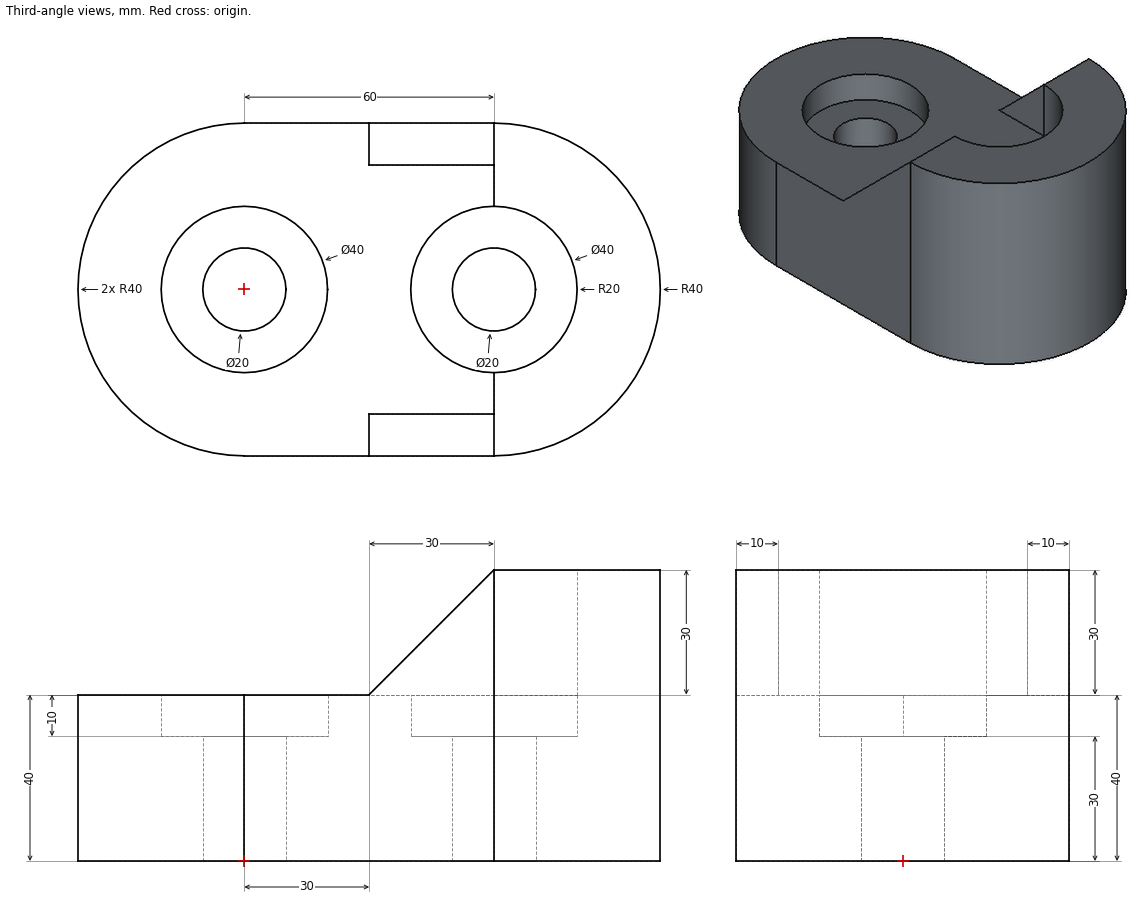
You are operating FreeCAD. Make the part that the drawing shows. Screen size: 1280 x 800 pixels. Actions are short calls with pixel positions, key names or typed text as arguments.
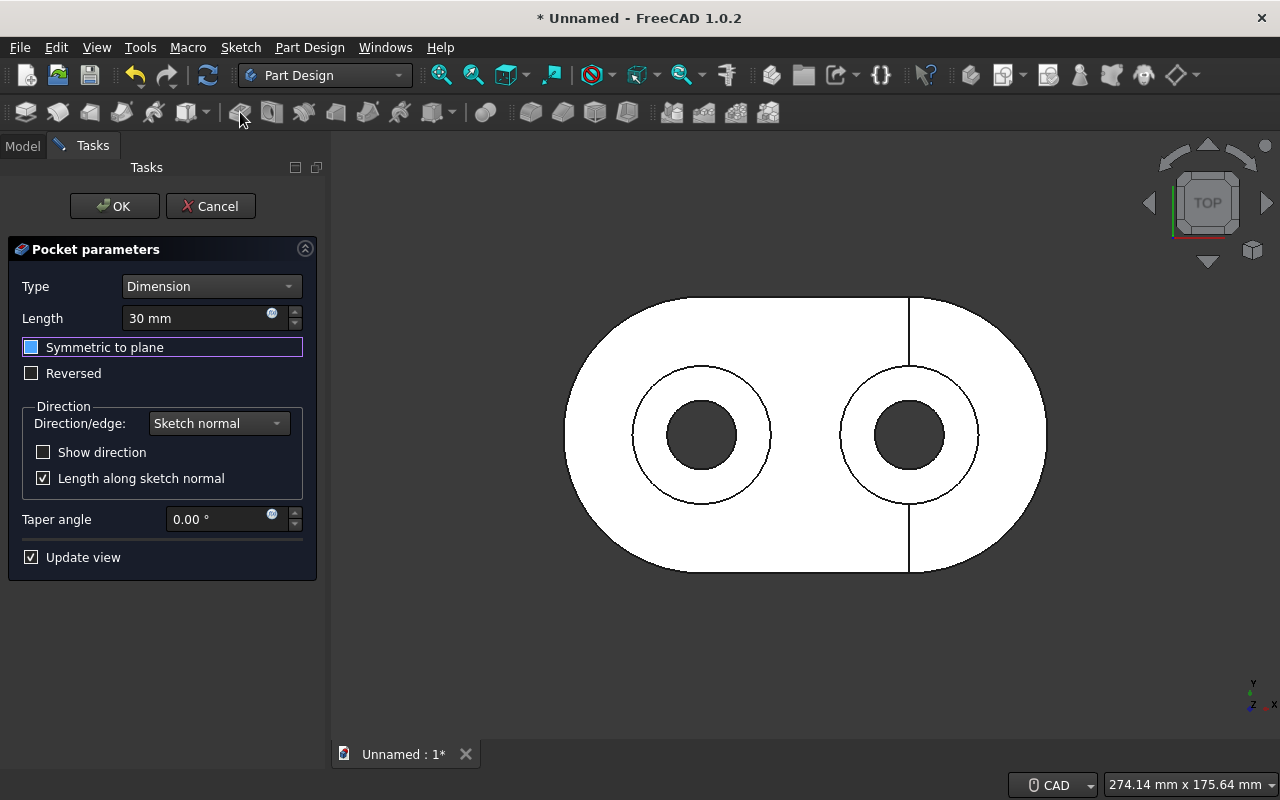
click(115, 206)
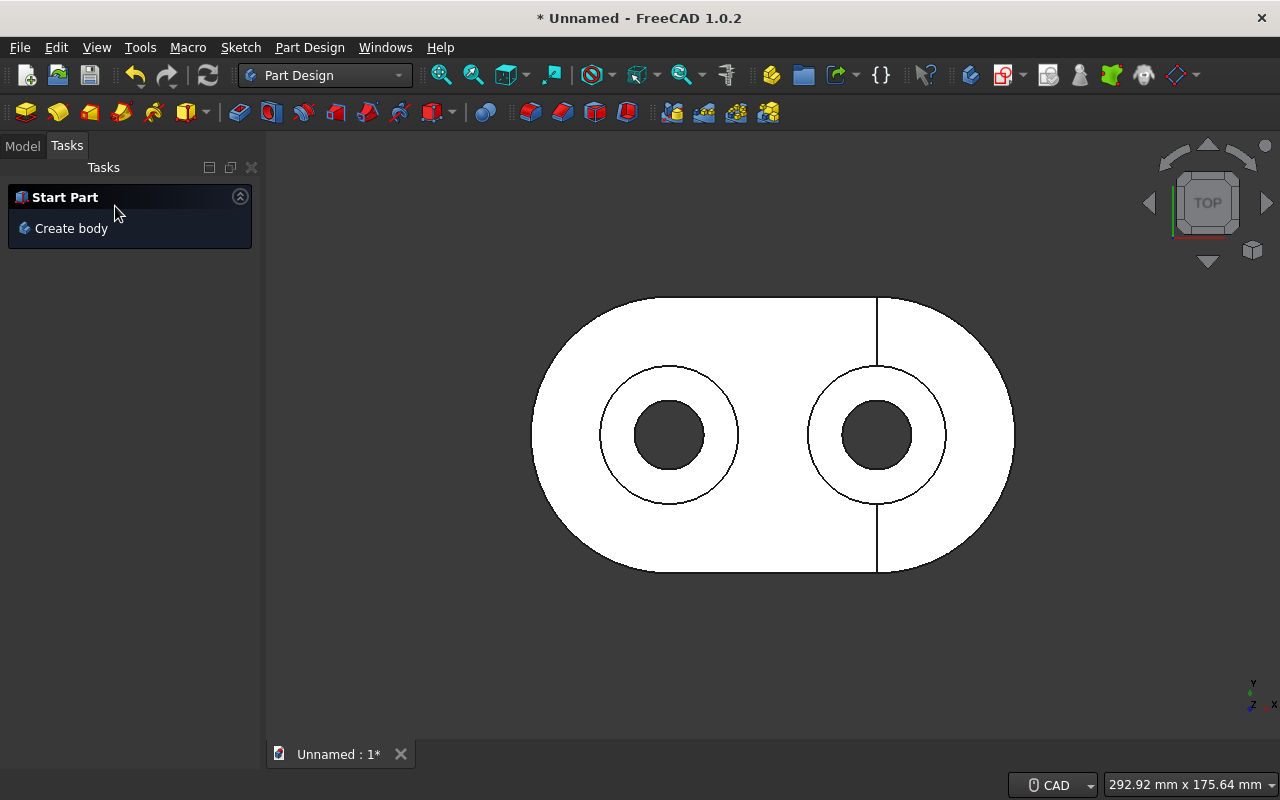
key(0)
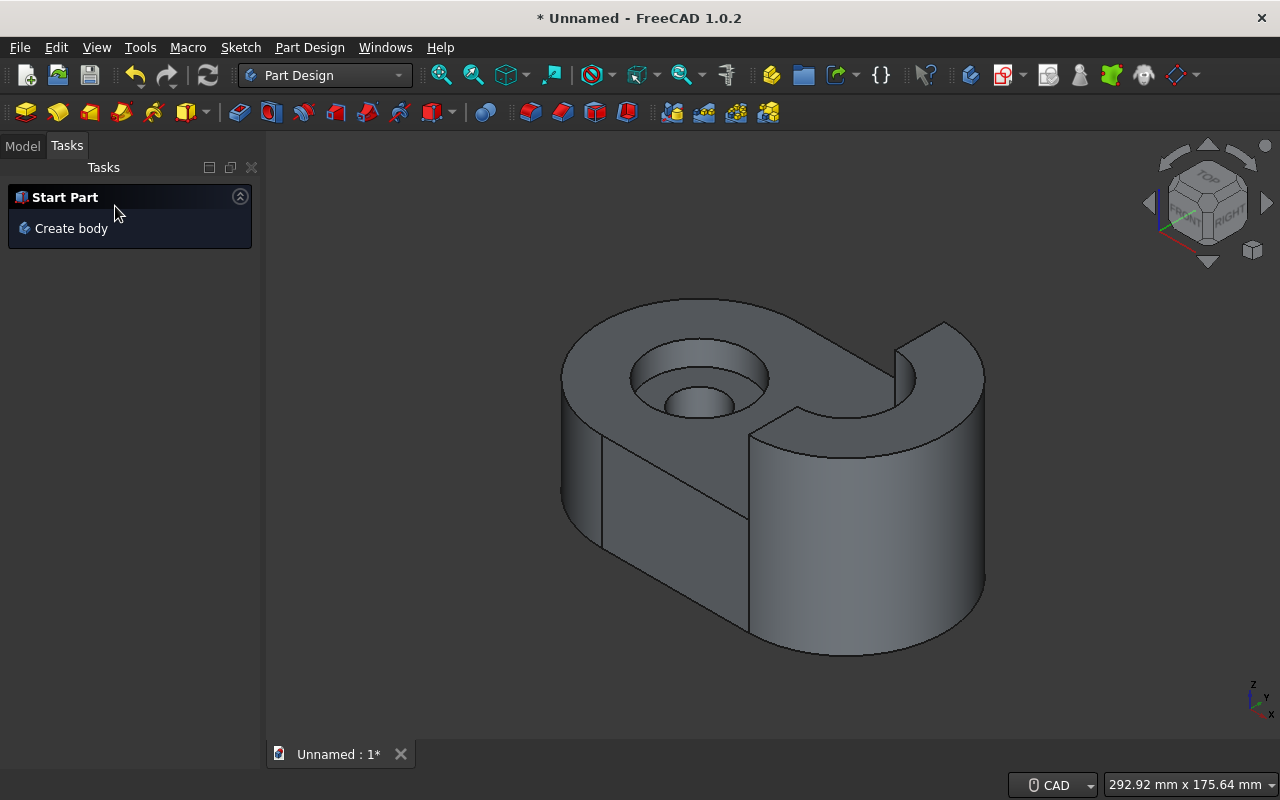
click(696, 545)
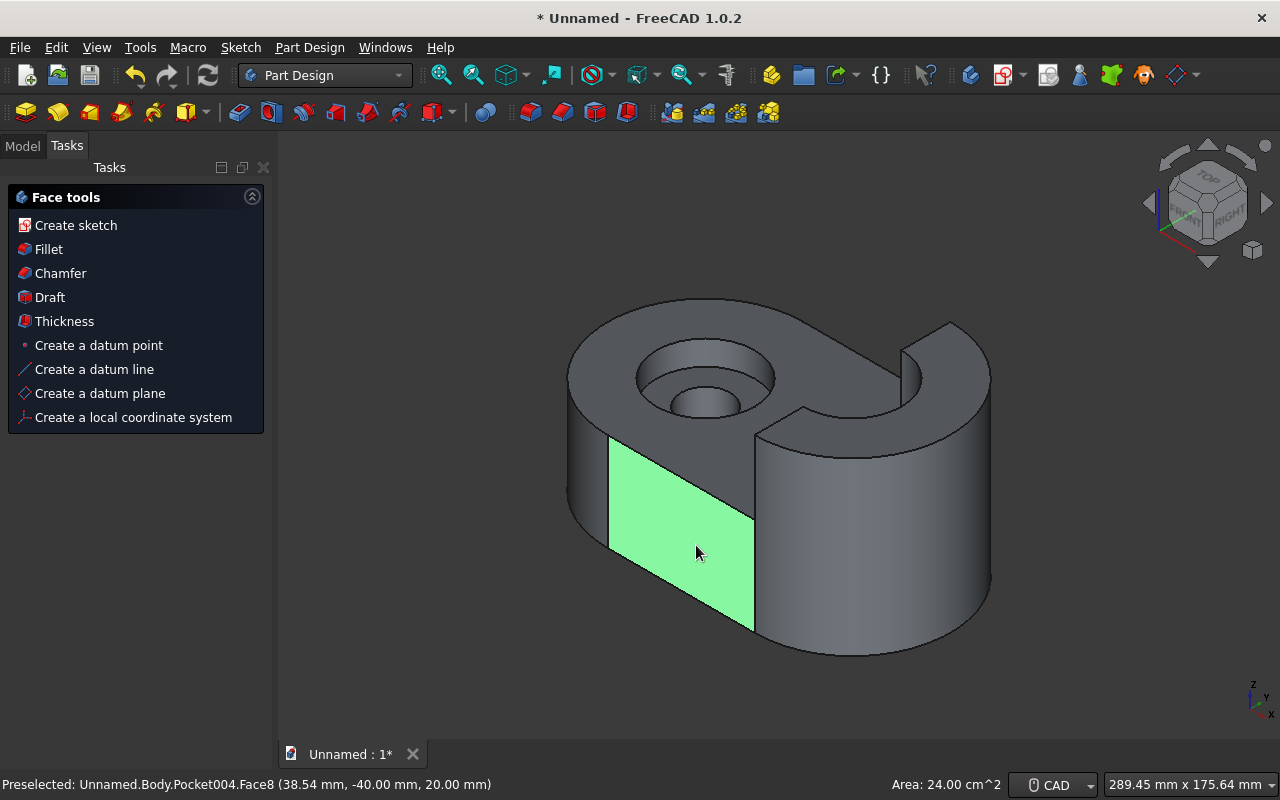
click(1004, 76)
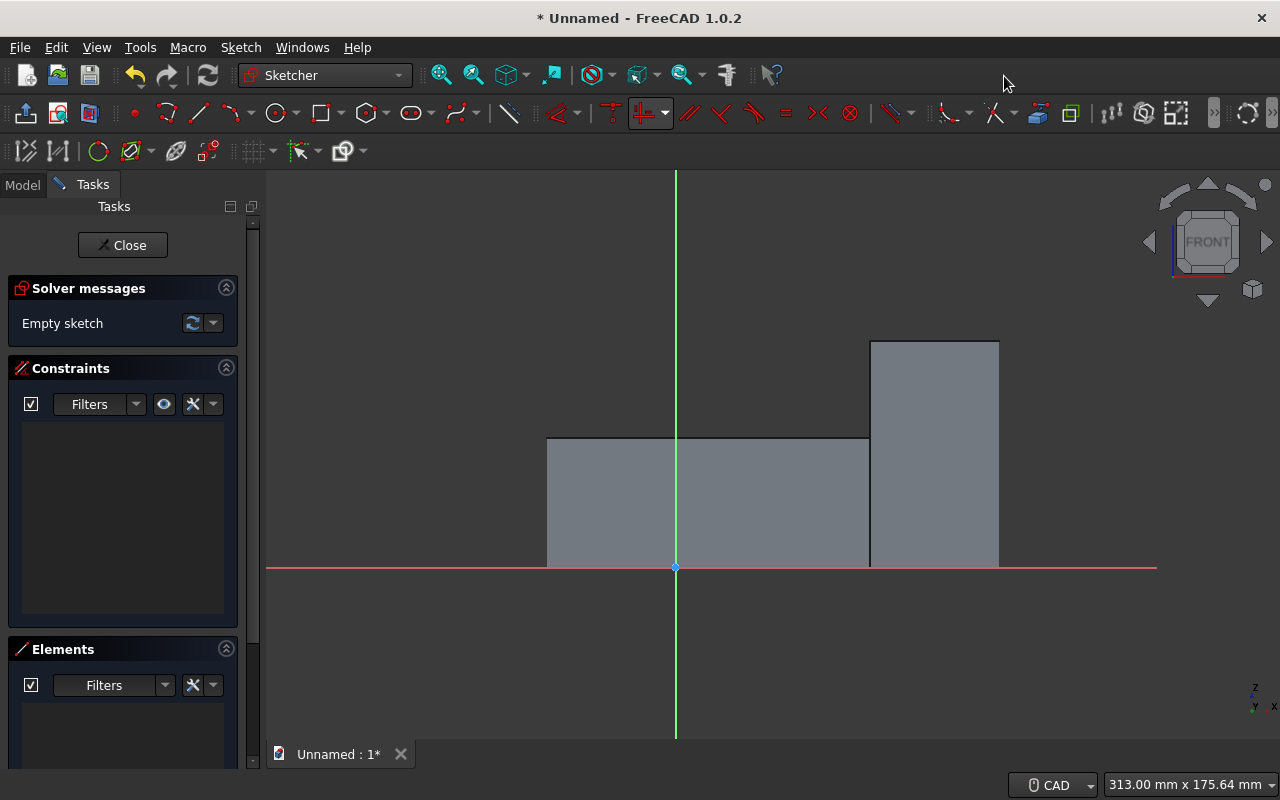
scroll(912, 454, up, 2)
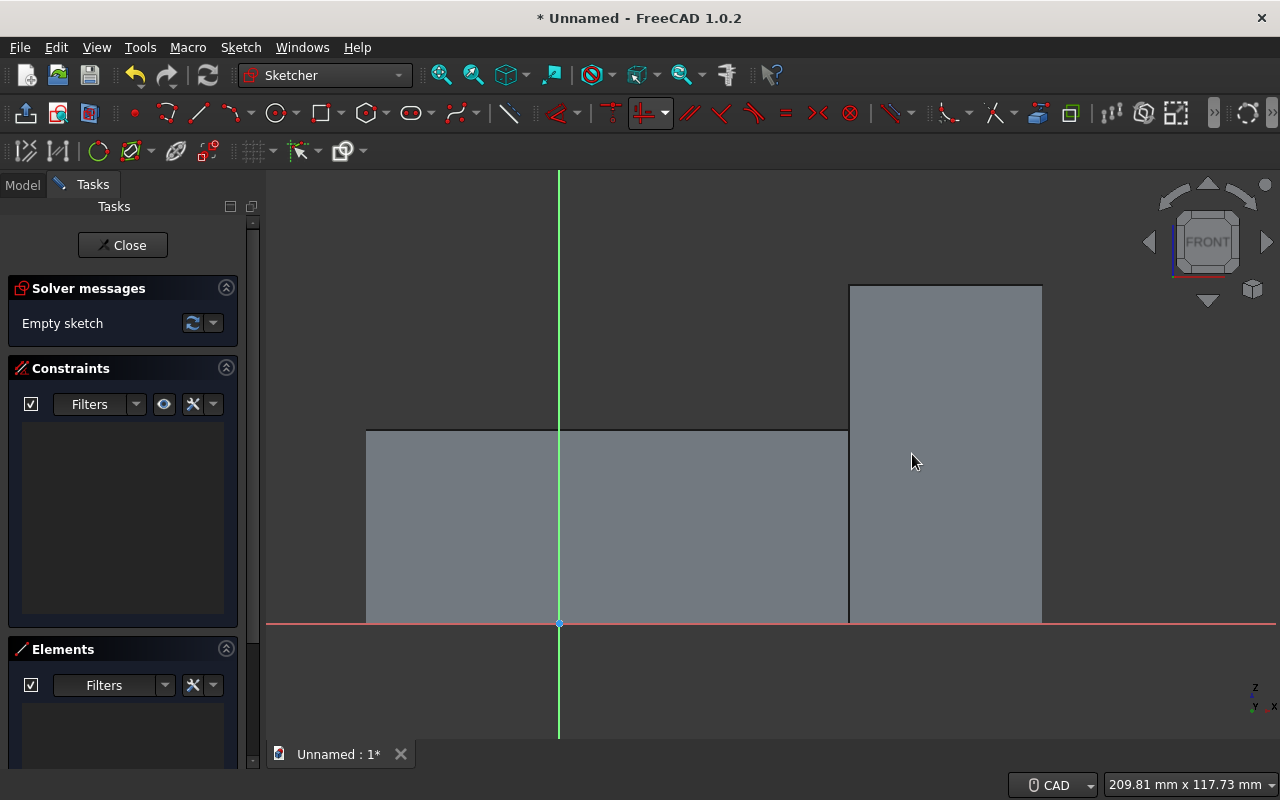
click(168, 114)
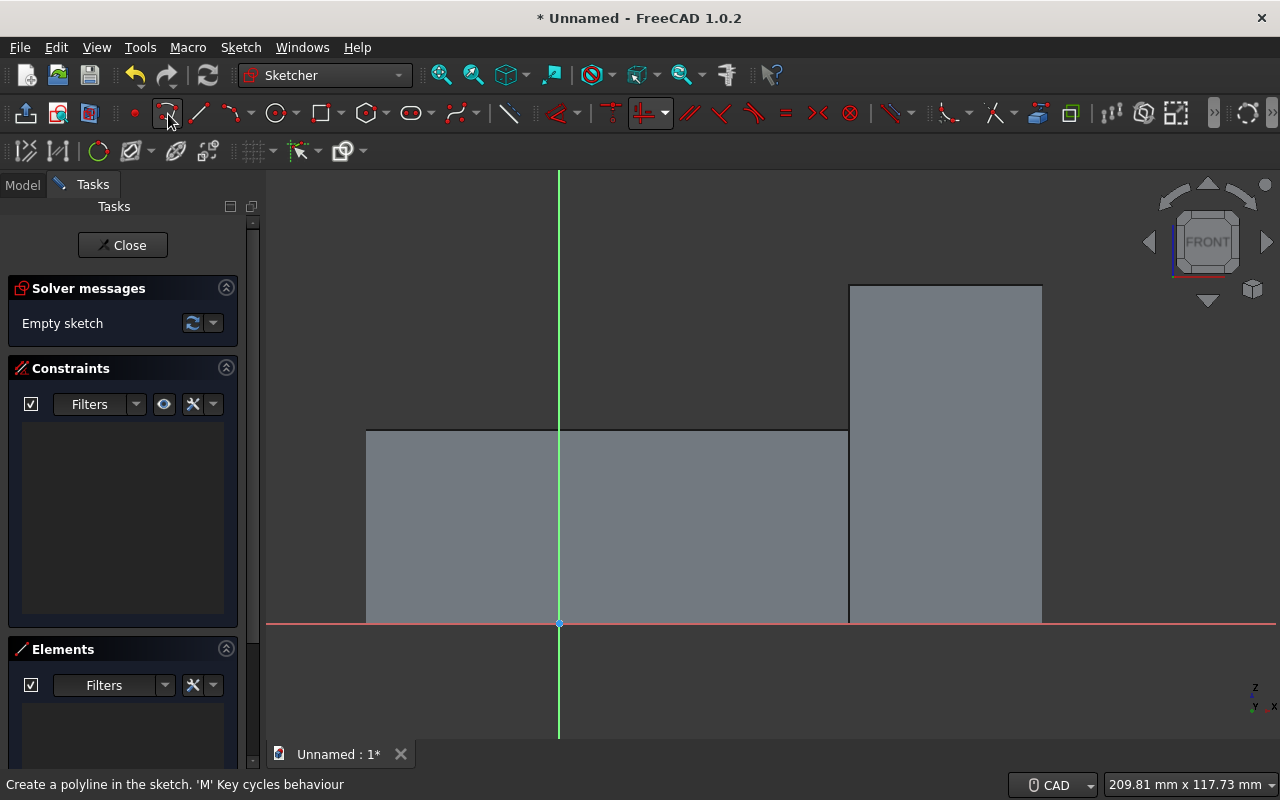
click(704, 430)
click(849, 430)
click(849, 285)
click(704, 431)
key(Escape)
key(Escape)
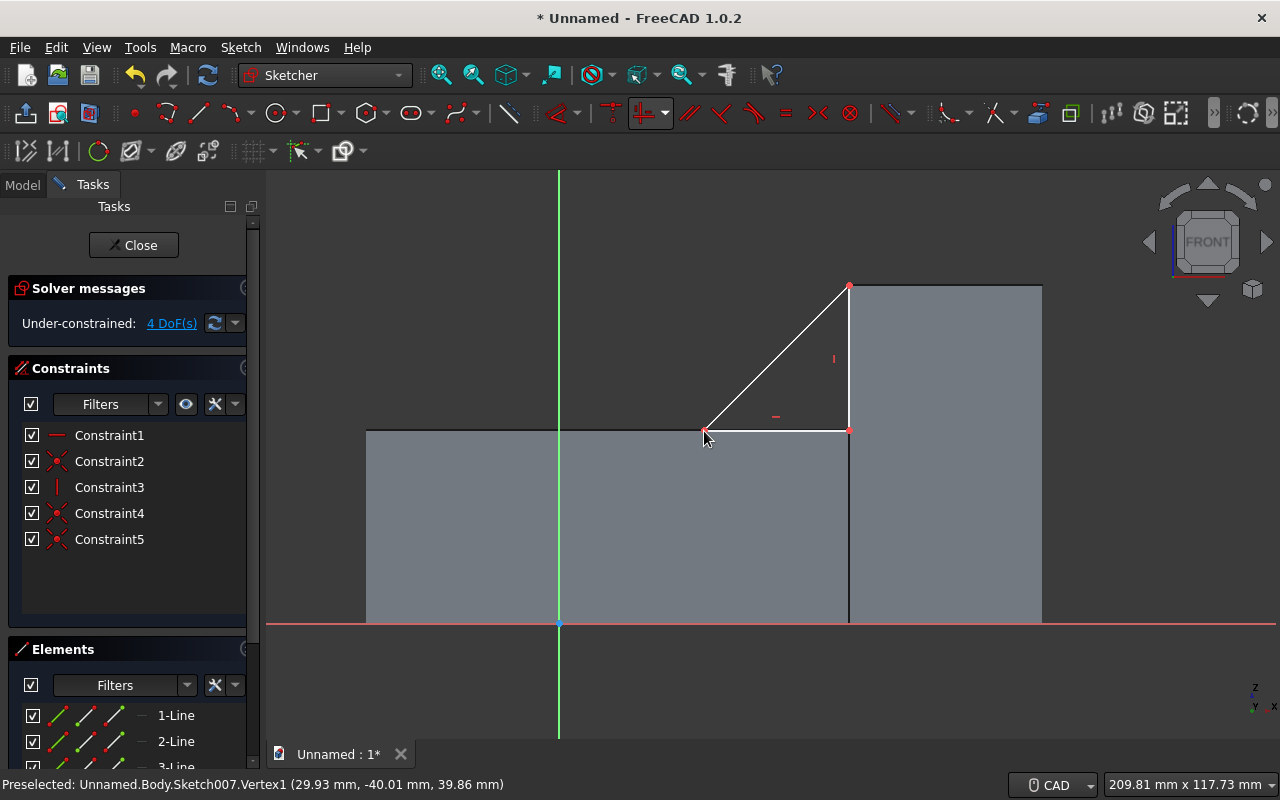
click(556, 114)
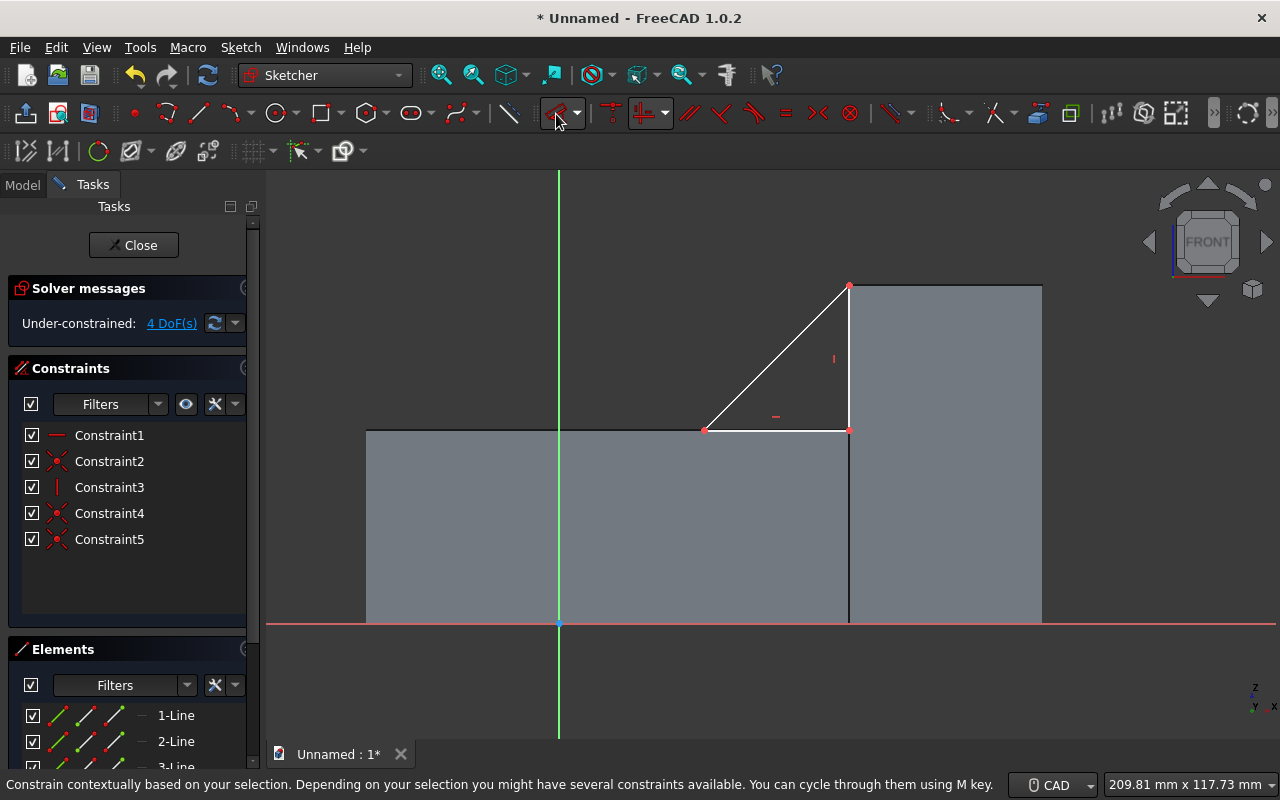
click(747, 431)
click(776, 397)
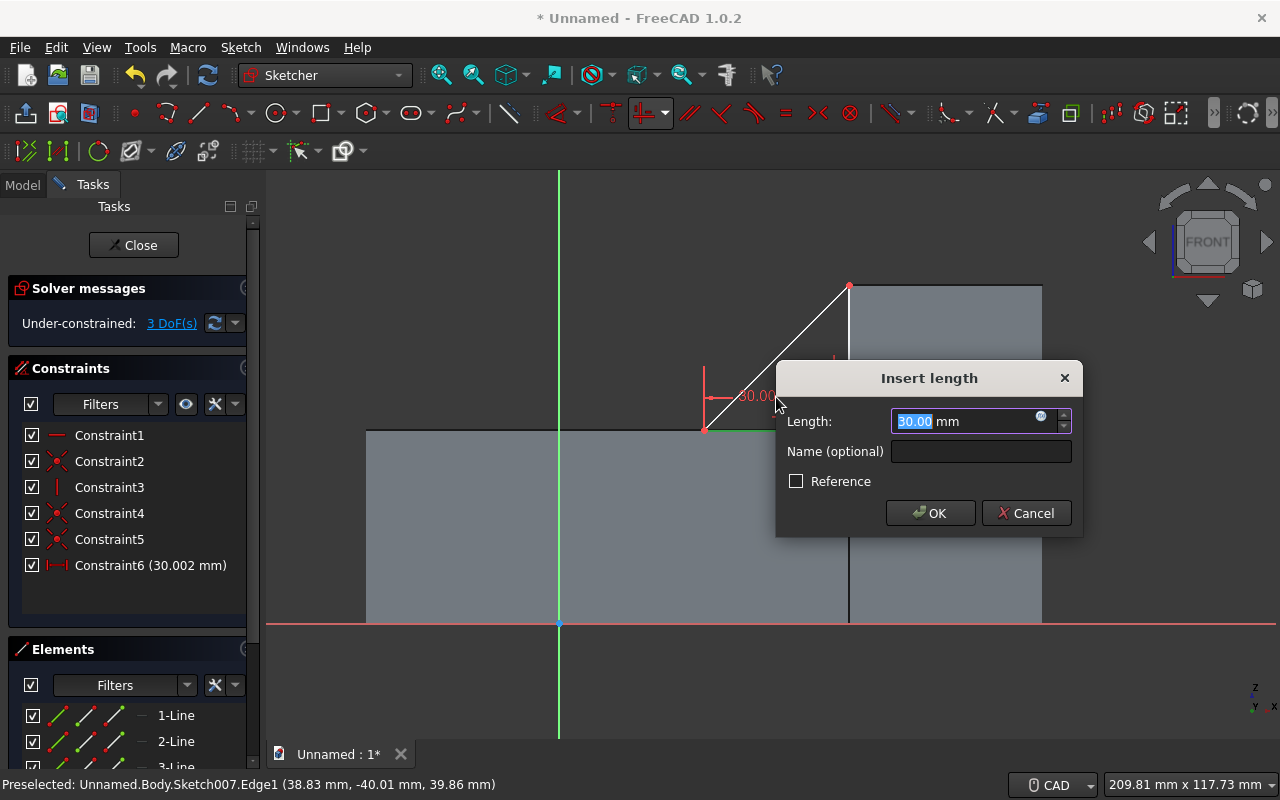
text(30)
key(Return)